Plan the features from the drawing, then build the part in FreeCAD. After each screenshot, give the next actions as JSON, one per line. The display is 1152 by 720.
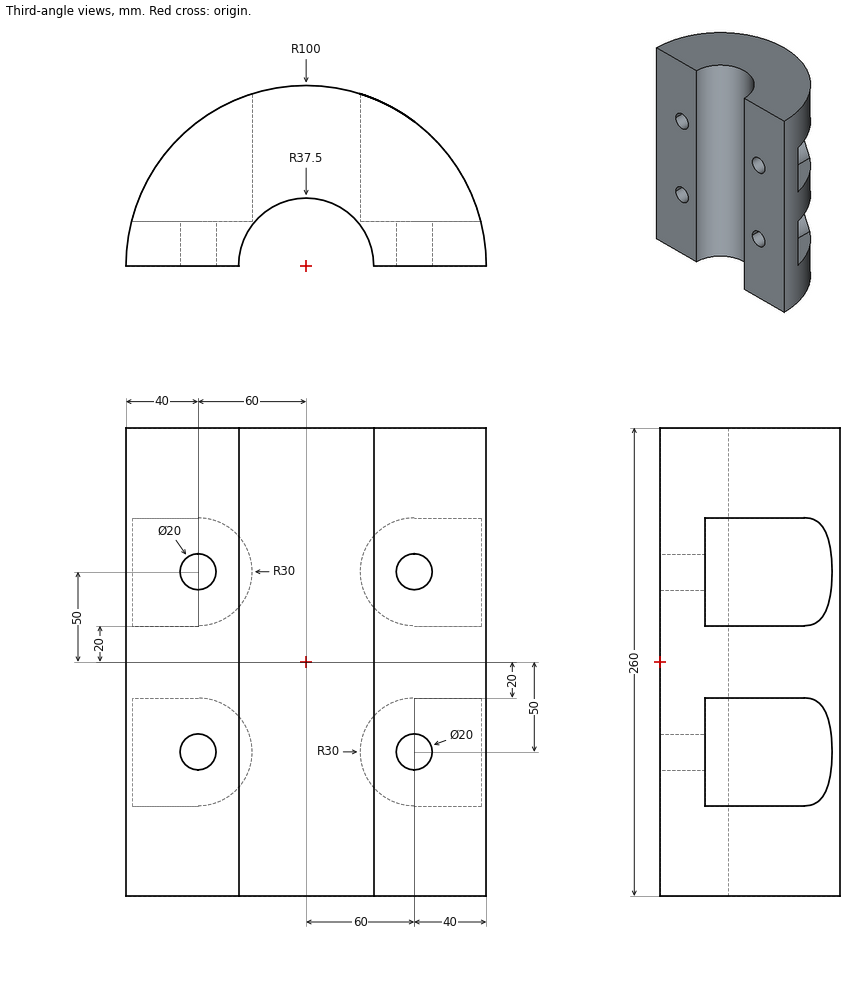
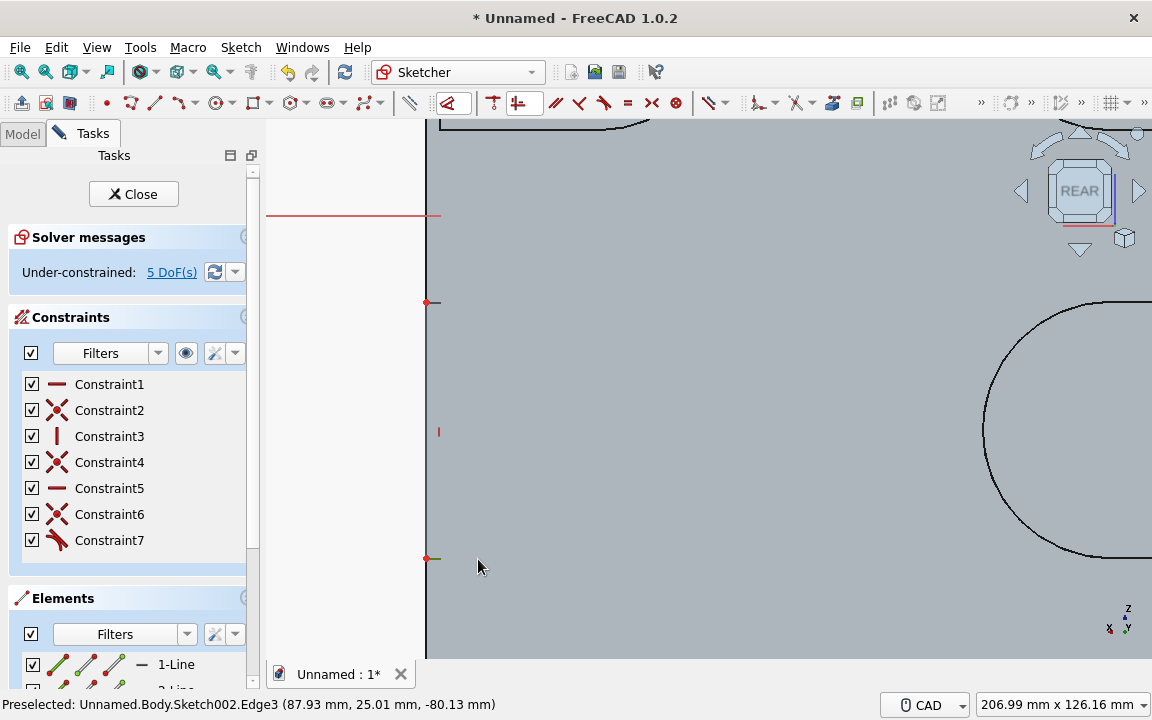
{"action": "left_click", "coordinate": [702, 506]}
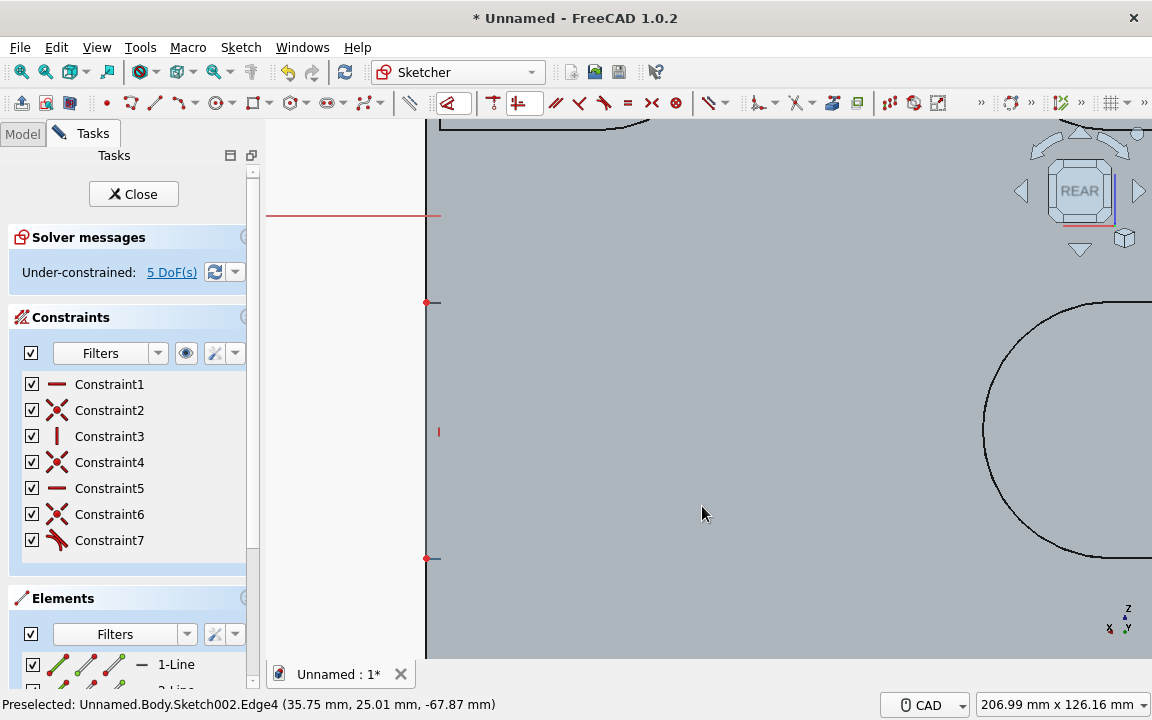
{"action": "key", "text": "t"}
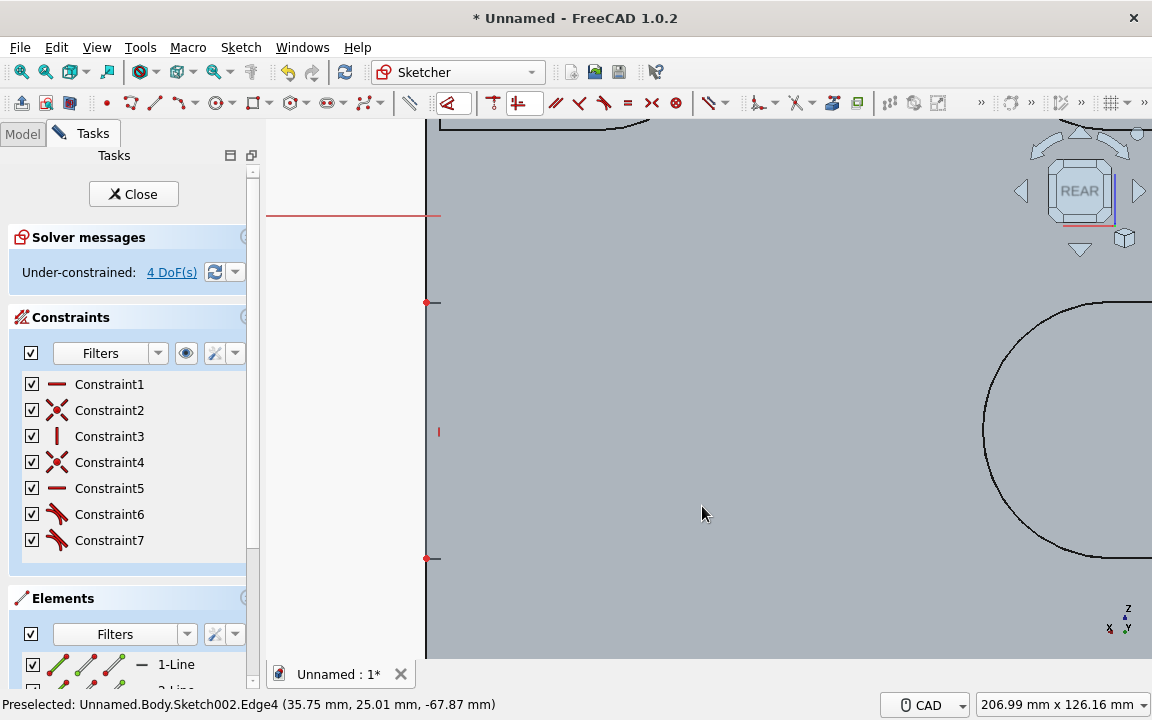
{"action": "left_click", "coordinate": [702, 506]}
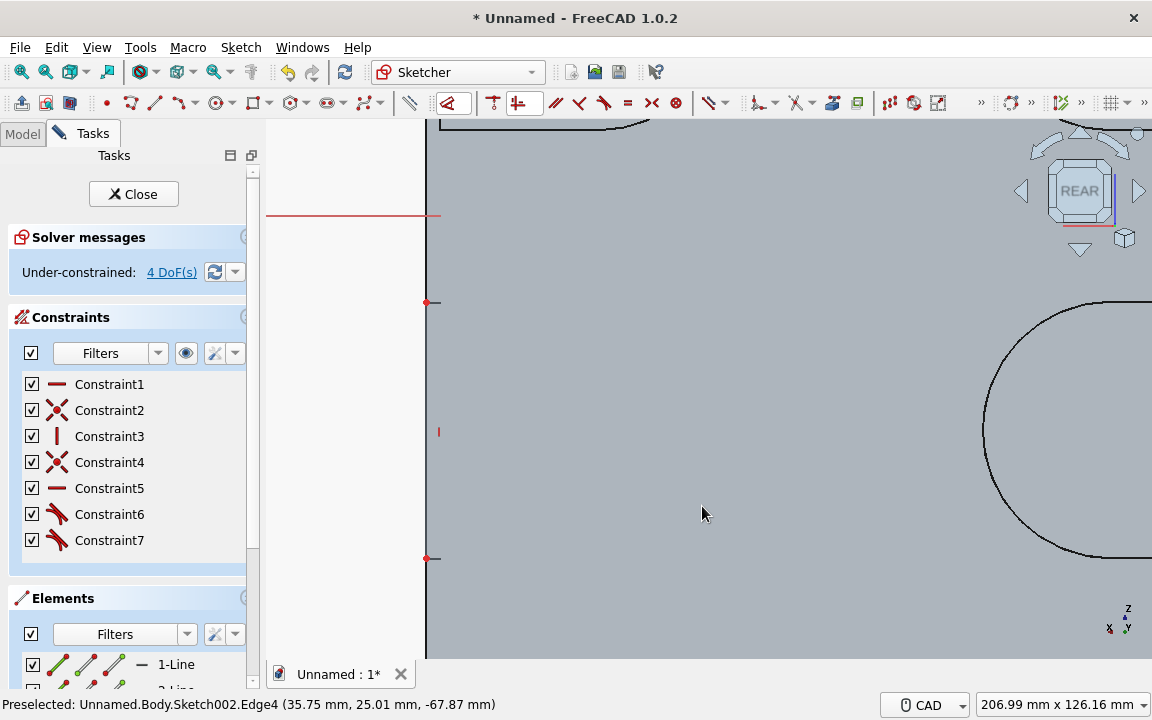
{"action": "left_click", "coordinate": [466, 104]}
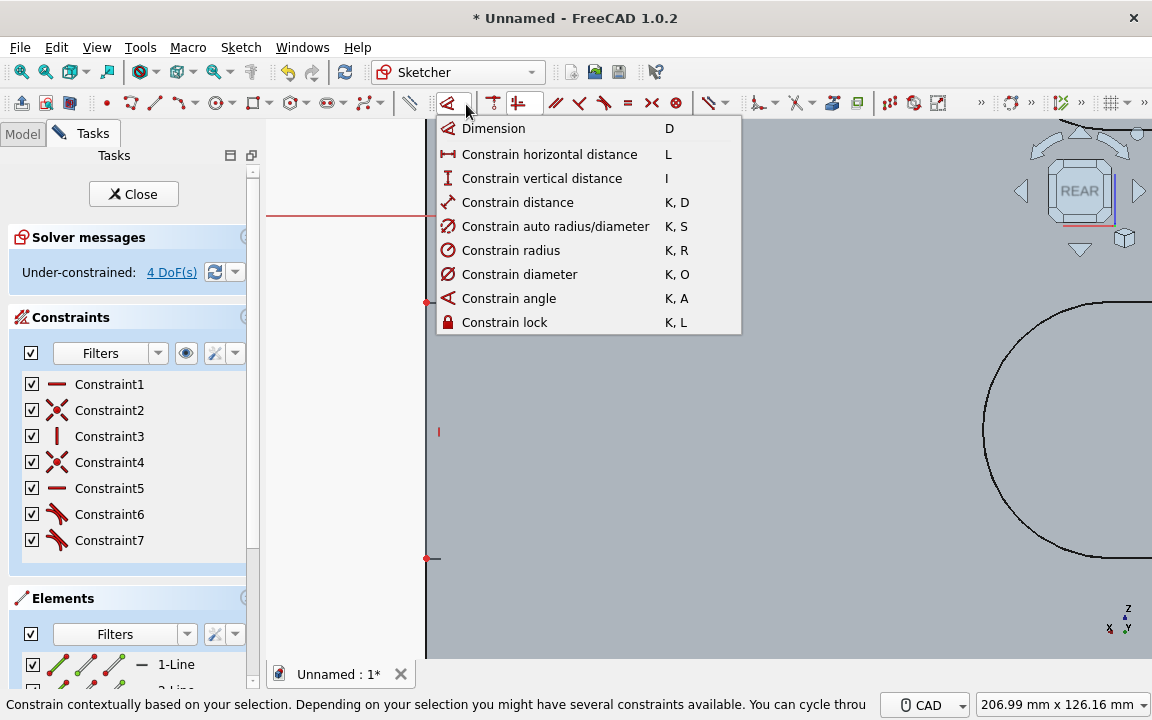
{"action": "left_click", "coordinate": [589, 250]}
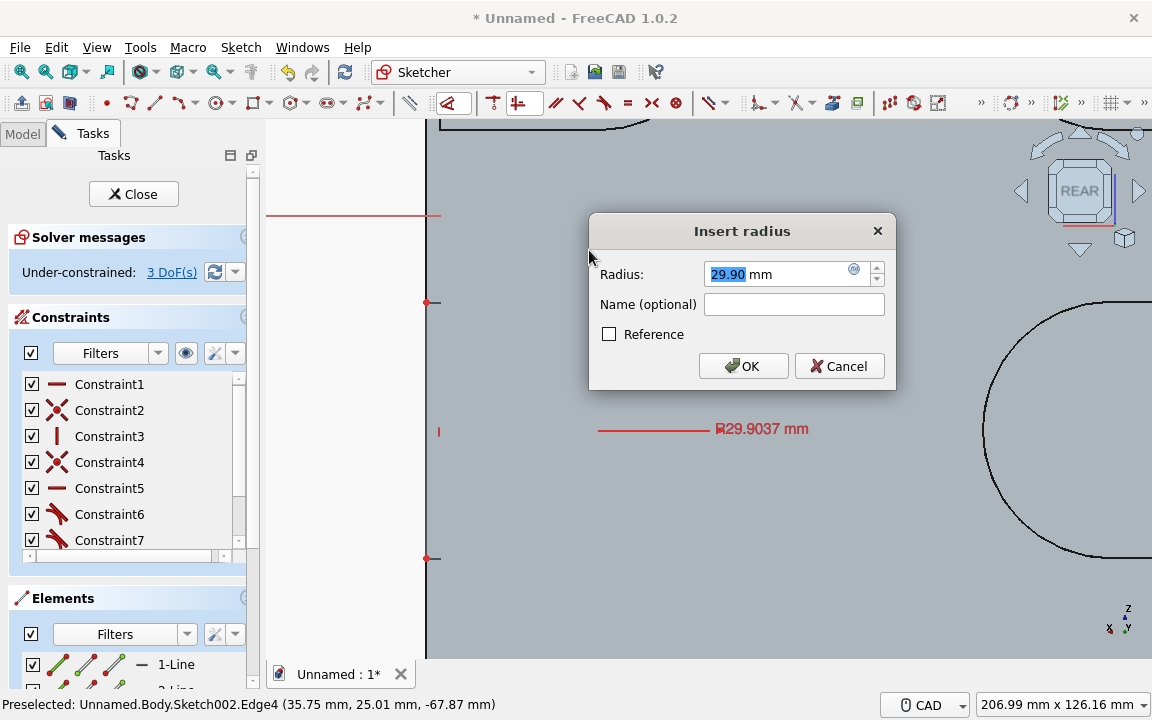
{"action": "type", "text": "30"}
{"action": "key", "text": "Return"}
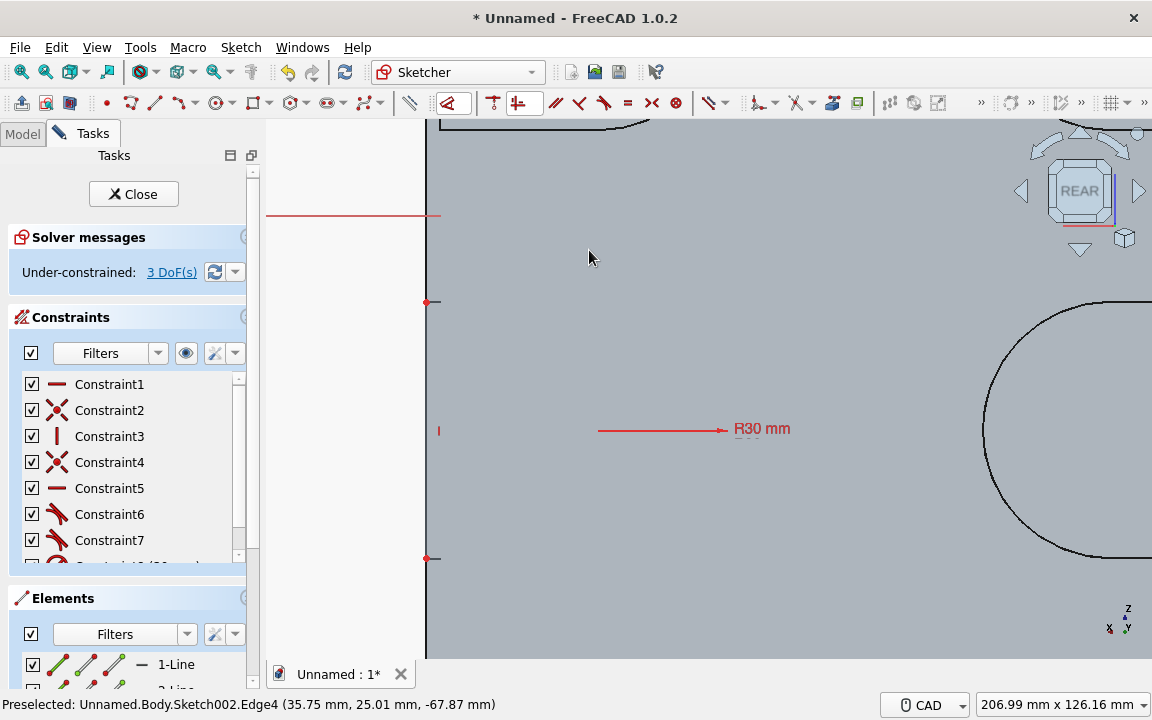
{"action": "left_click", "coordinate": [546, 302]}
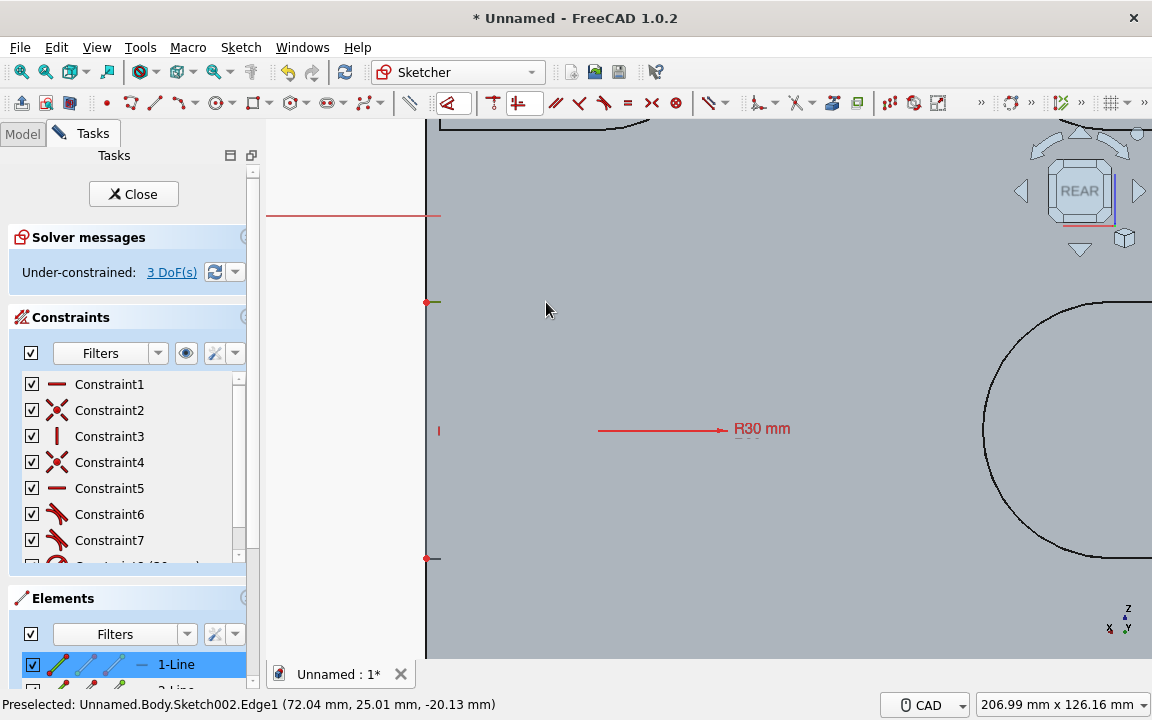
{"action": "left_click", "coordinate": [466, 104]}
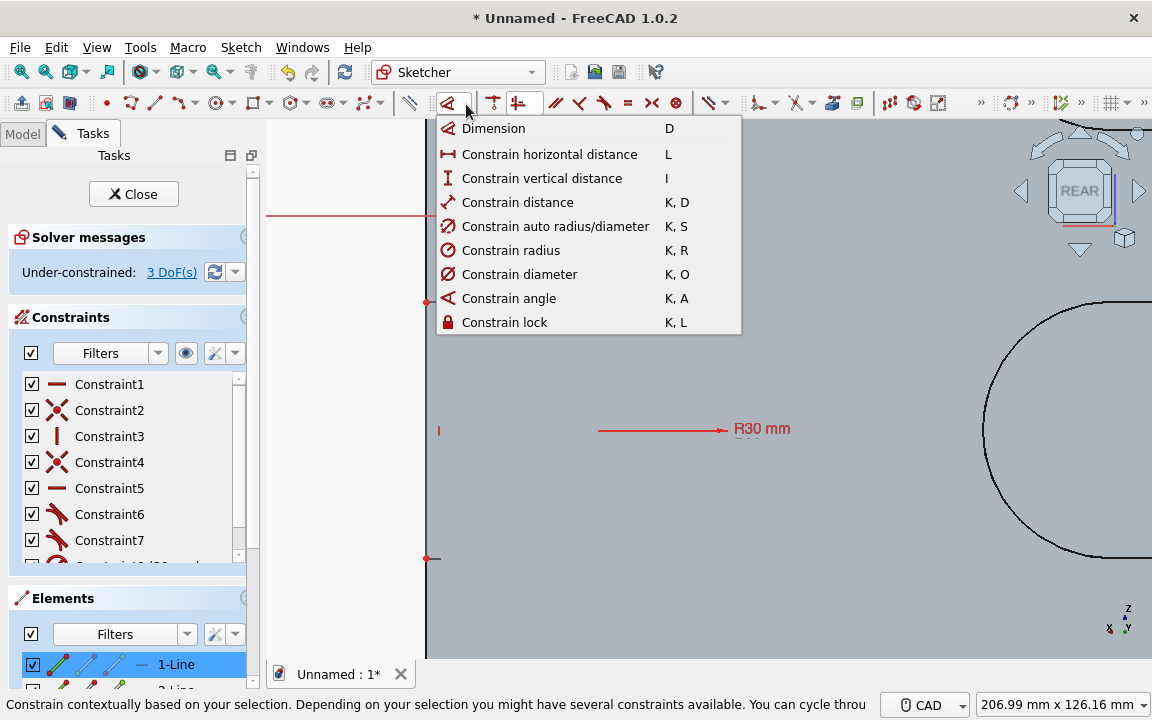
{"action": "left_click", "coordinate": [589, 154]}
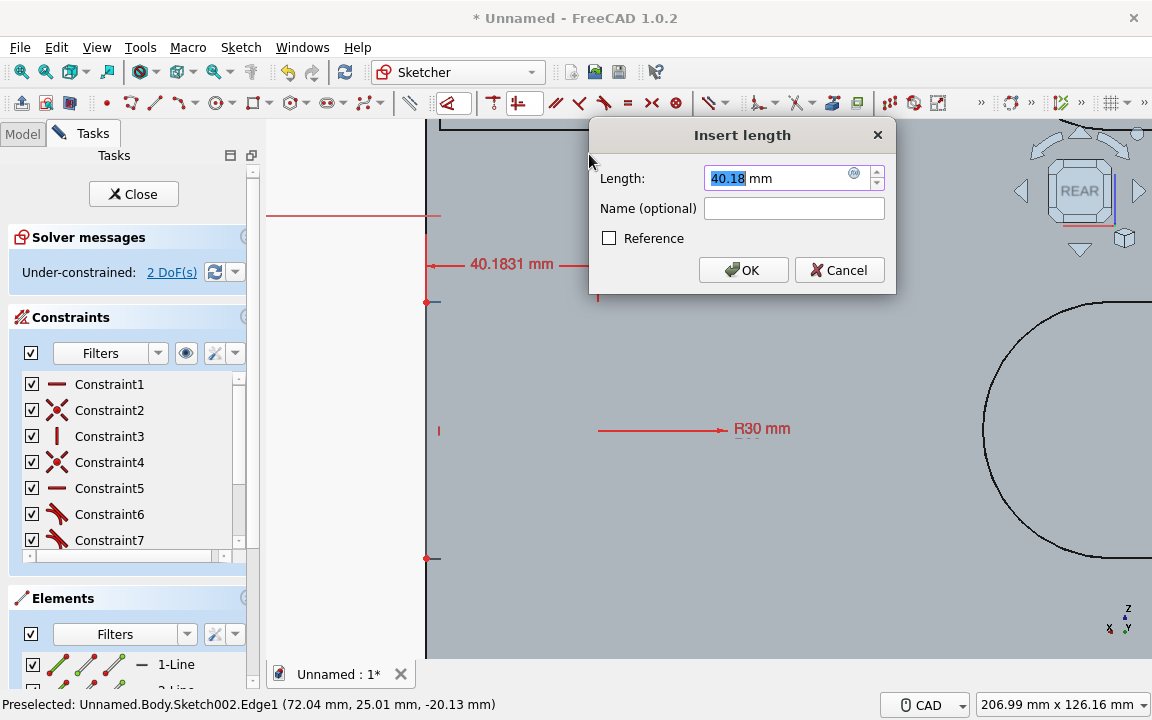
{"action": "type", "text": "40"}
{"action": "key", "text": "Return"}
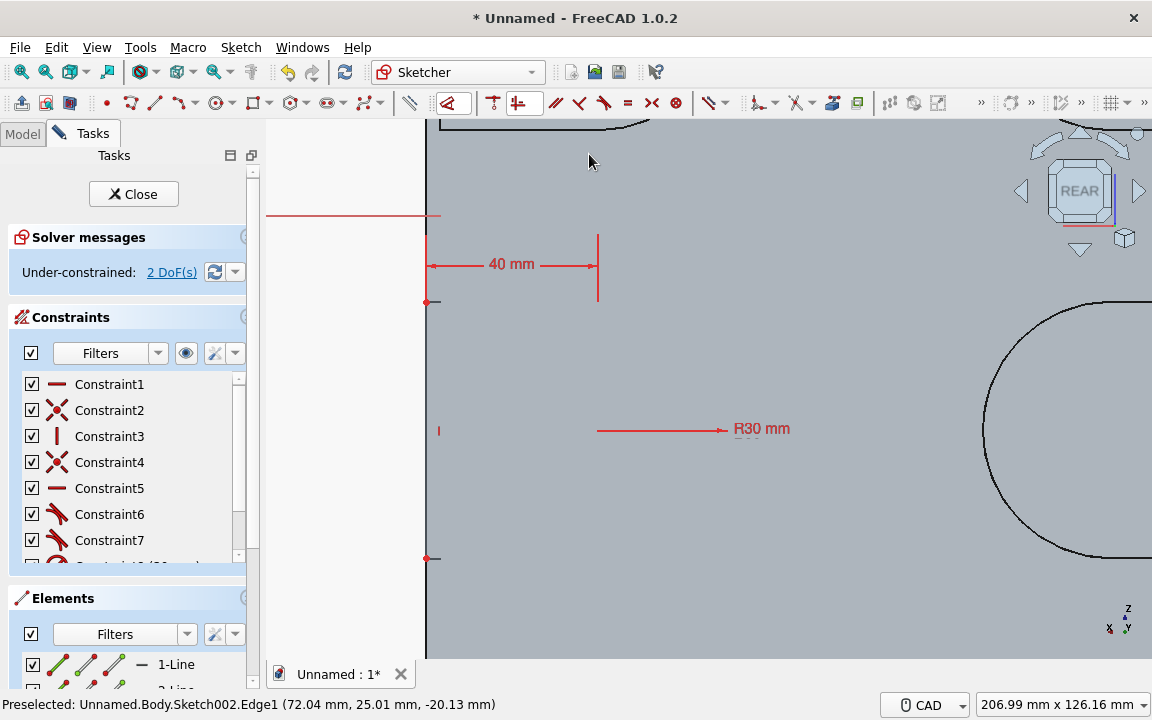
{"action": "left_click", "coordinate": [598, 302]}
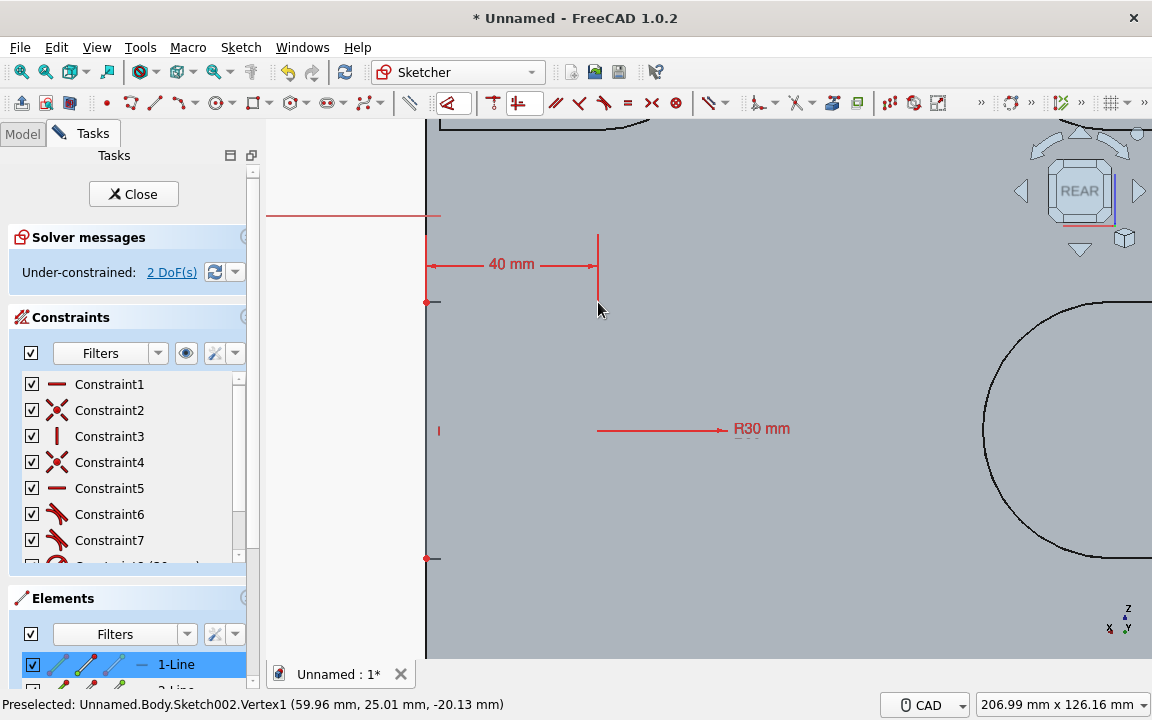
{"action": "key", "text": "l"}